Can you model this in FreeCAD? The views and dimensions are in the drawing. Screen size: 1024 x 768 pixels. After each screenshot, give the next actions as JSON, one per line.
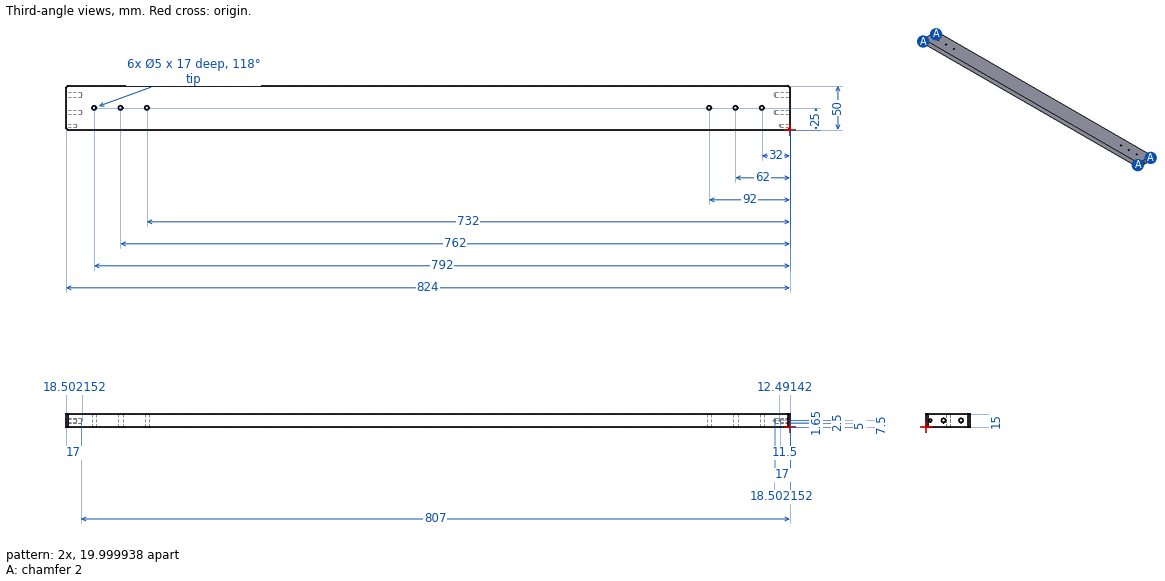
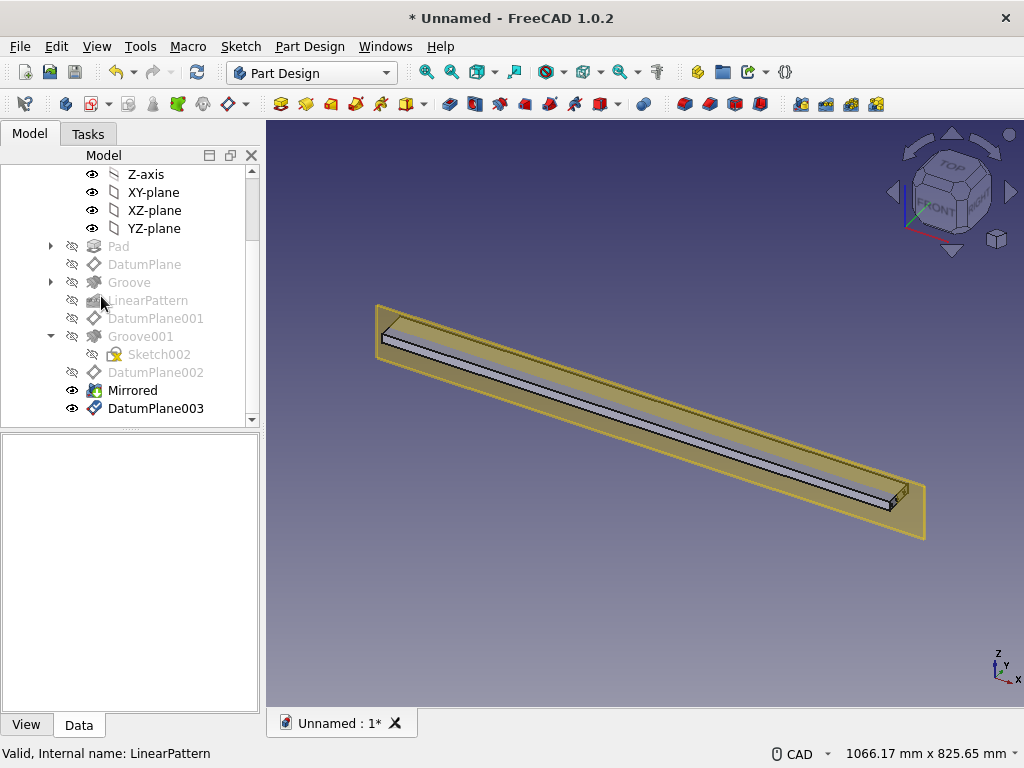
{"action": "left_click", "coordinate": [117, 408]}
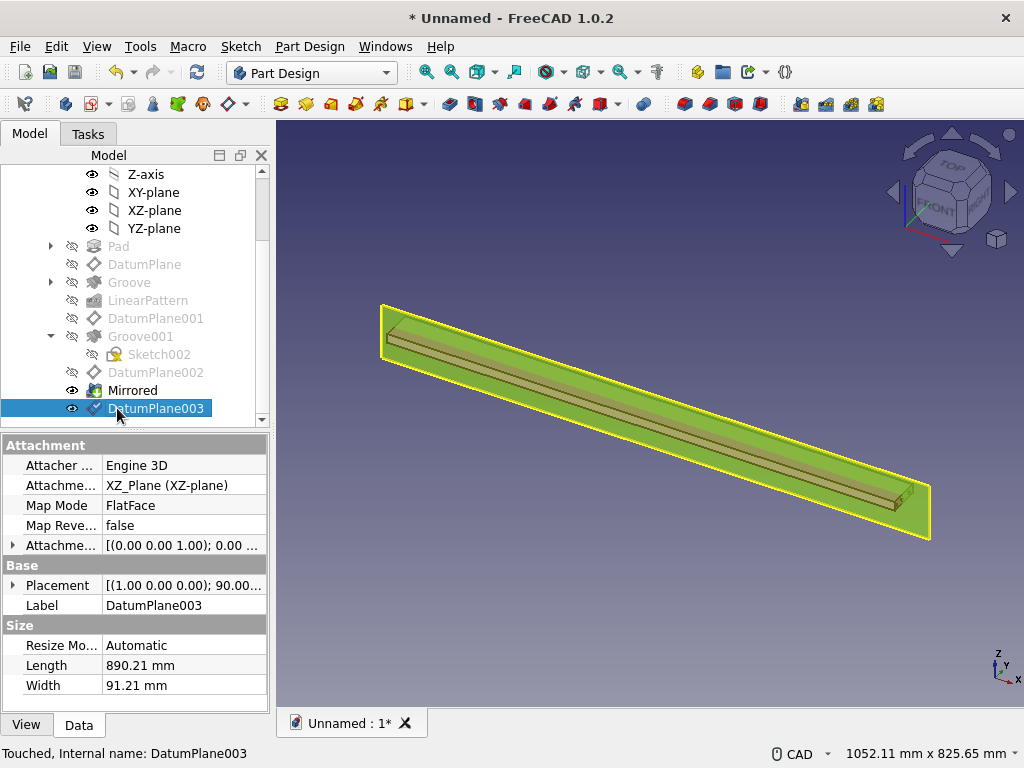
{"action": "left_click", "coordinate": [90, 104]}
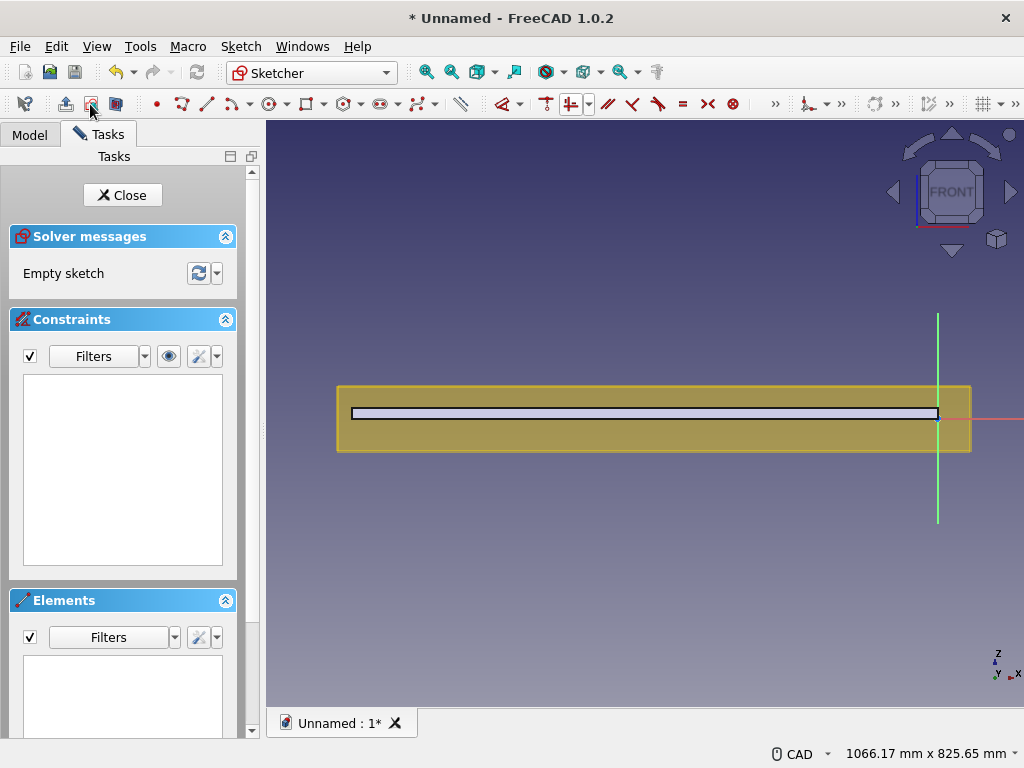
{"action": "left_click", "coordinate": [116, 104]}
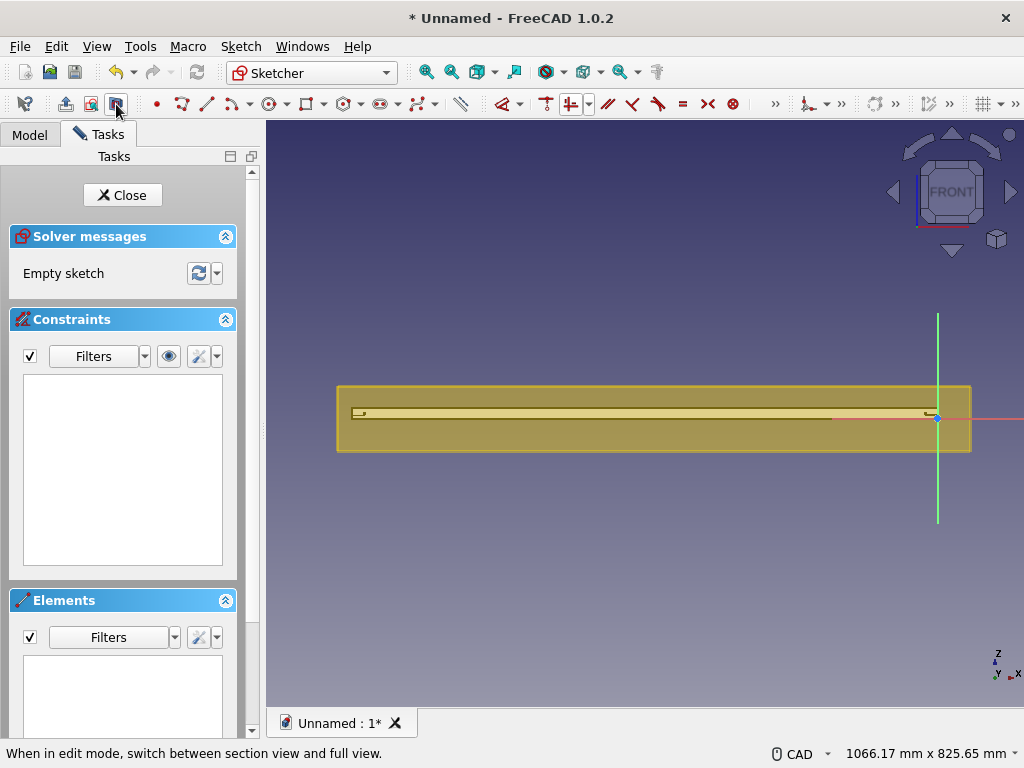
{"action": "scroll", "coordinate": [344, 414], "scroll_direction": "up", "scroll_amount": 15}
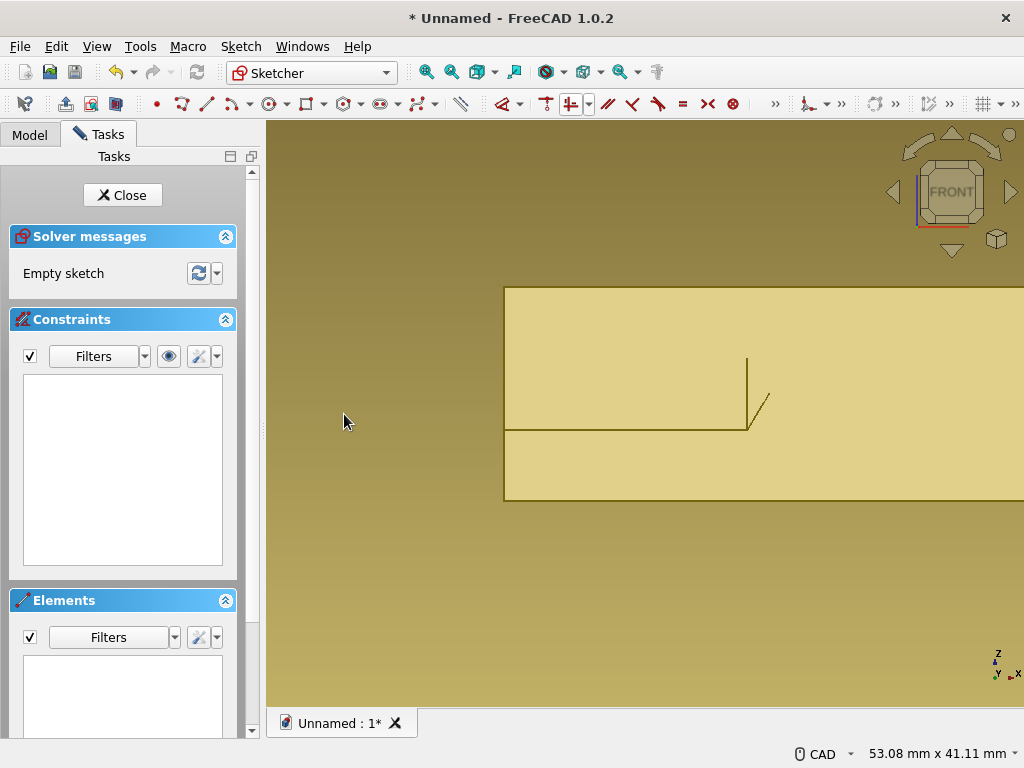
{"action": "left_click", "coordinate": [182, 104]}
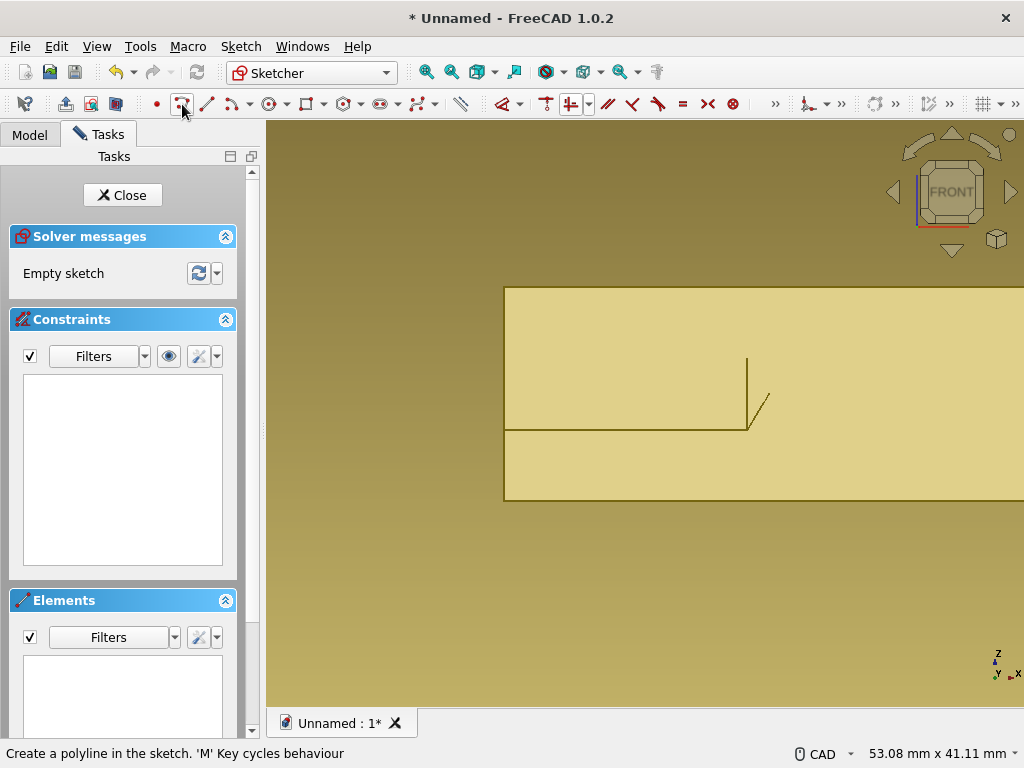
{"action": "left_click", "coordinate": [769, 394]}
{"action": "left_click", "coordinate": [747, 430]}
{"action": "left_click", "coordinate": [504, 430]}
{"action": "left_click", "coordinate": [504, 394]}
{"action": "left_click", "coordinate": [769, 395]}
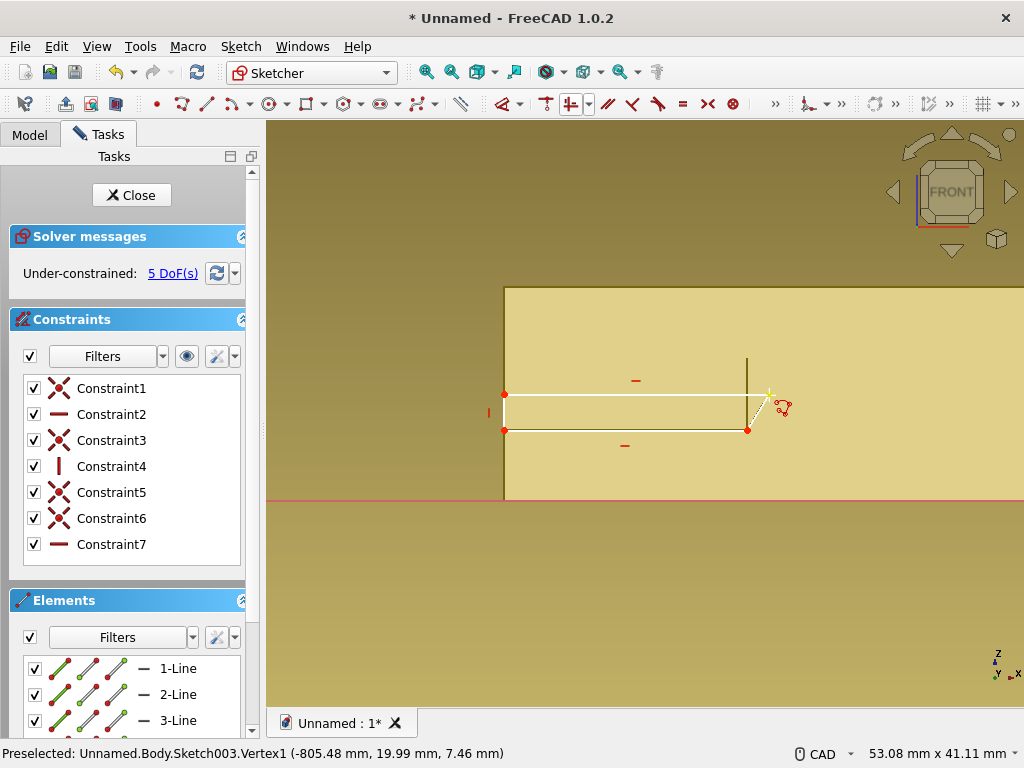
{"action": "left_click", "coordinate": [207, 104]}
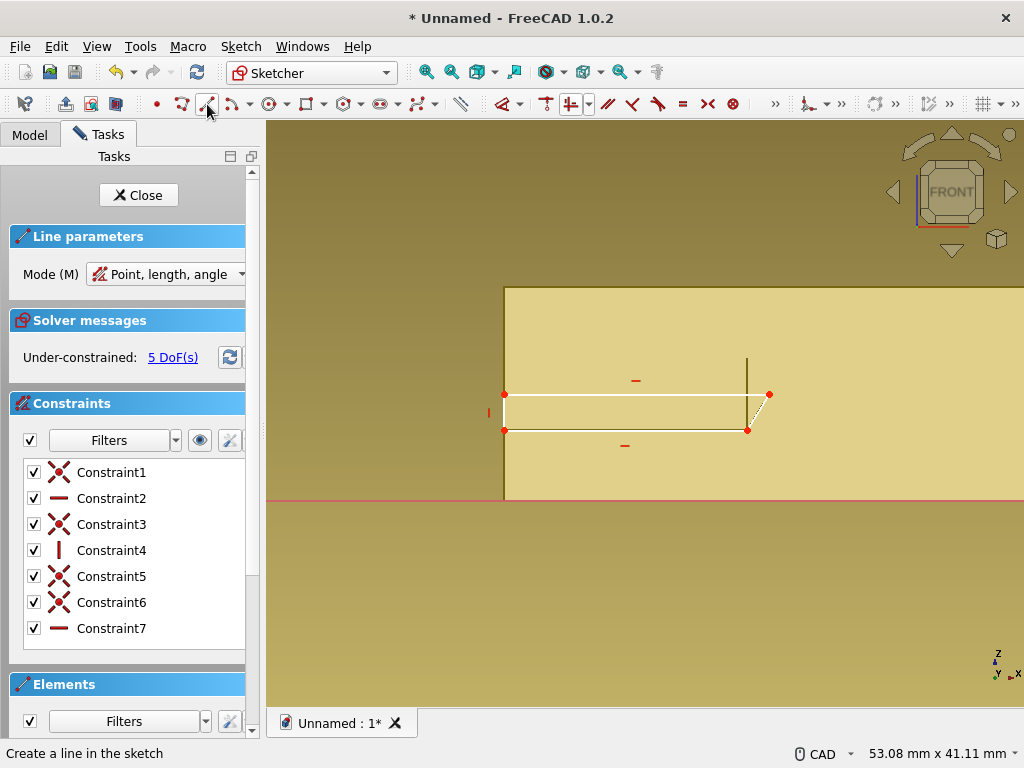
{"action": "left_click", "coordinate": [478, 394]}
{"action": "left_click", "coordinate": [399, 394]}
{"action": "key", "text": "Escape"}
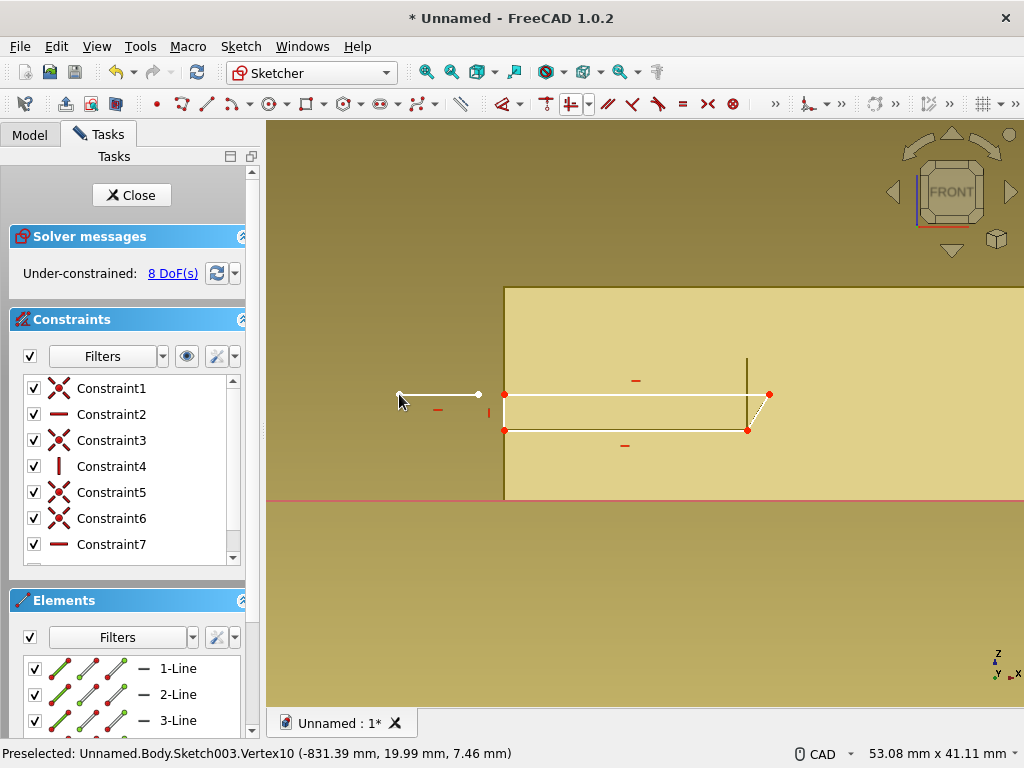
{"action": "left_click", "coordinate": [454, 395]}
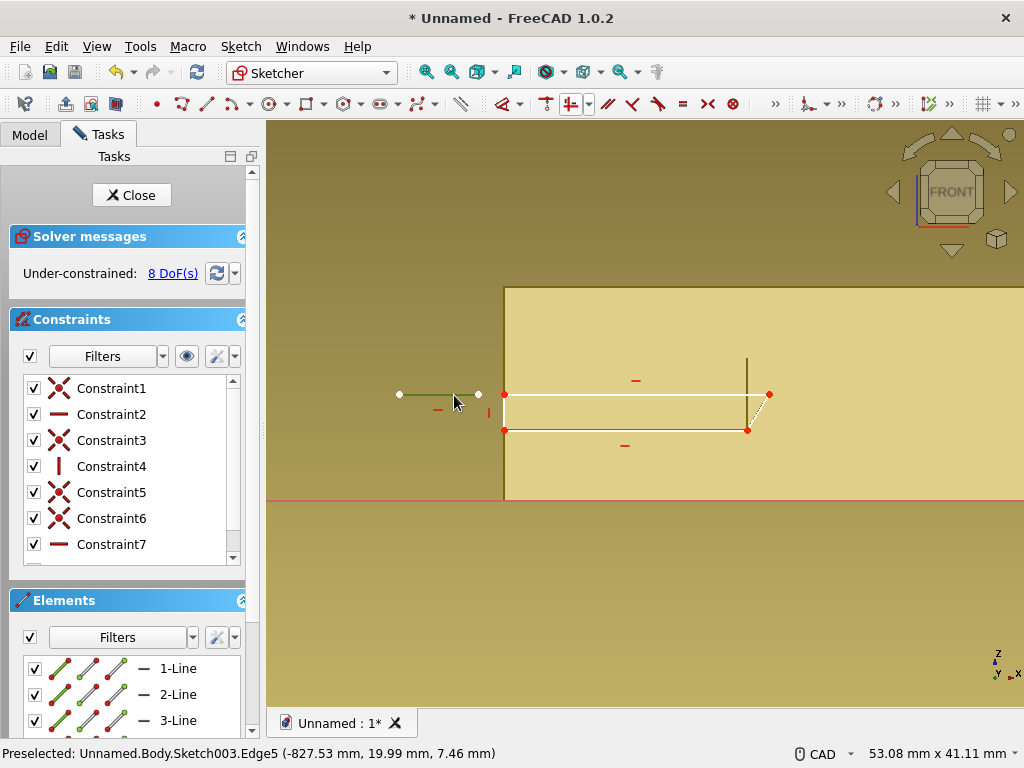
{"action": "left_click", "coordinate": [461, 104]}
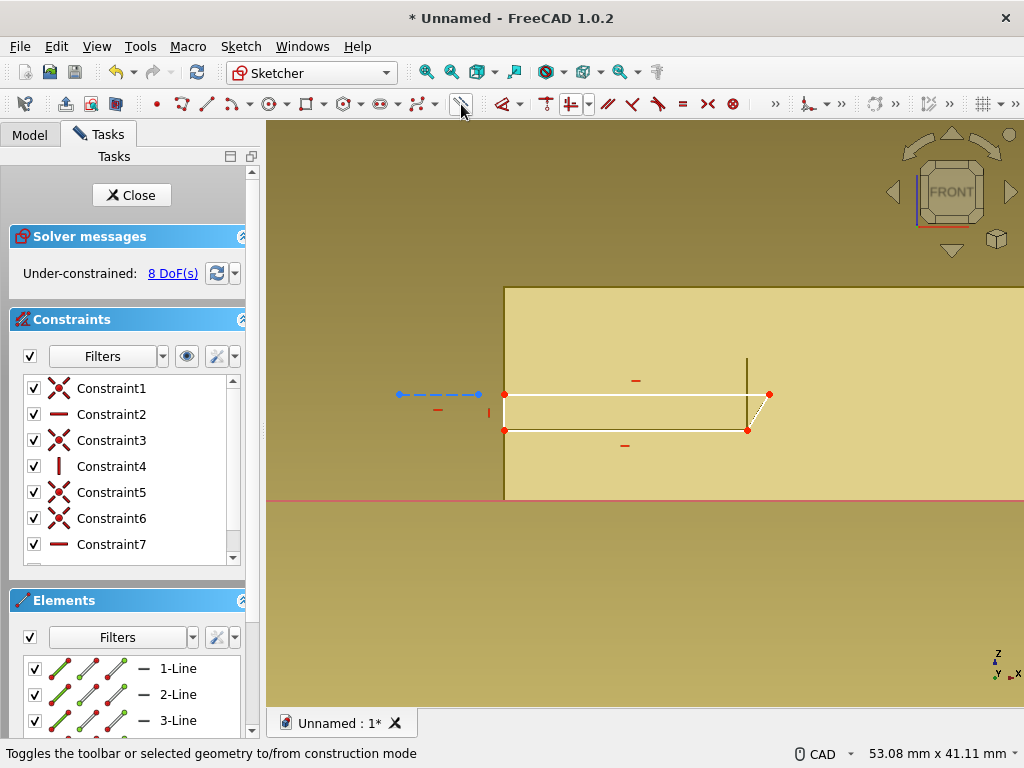
{"action": "left_click", "coordinate": [502, 104]}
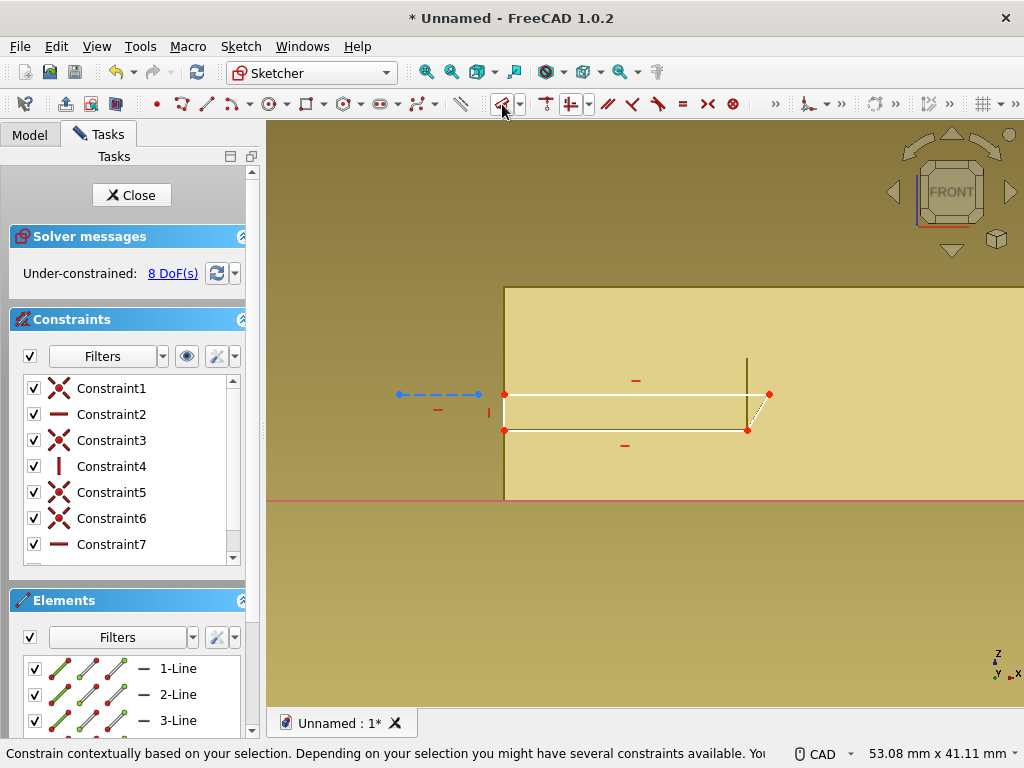
{"action": "left_click", "coordinate": [674, 431]}
{"action": "left_click", "coordinate": [626, 465]}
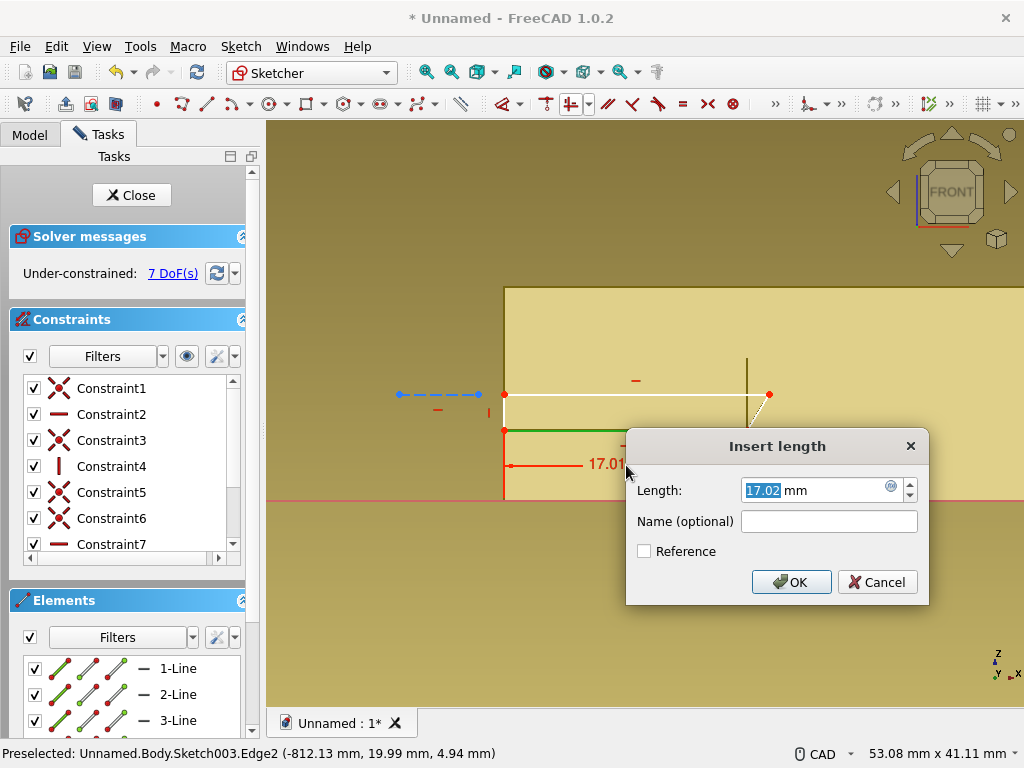
{"action": "type", "text": "17"}
{"action": "key", "text": "Return"}